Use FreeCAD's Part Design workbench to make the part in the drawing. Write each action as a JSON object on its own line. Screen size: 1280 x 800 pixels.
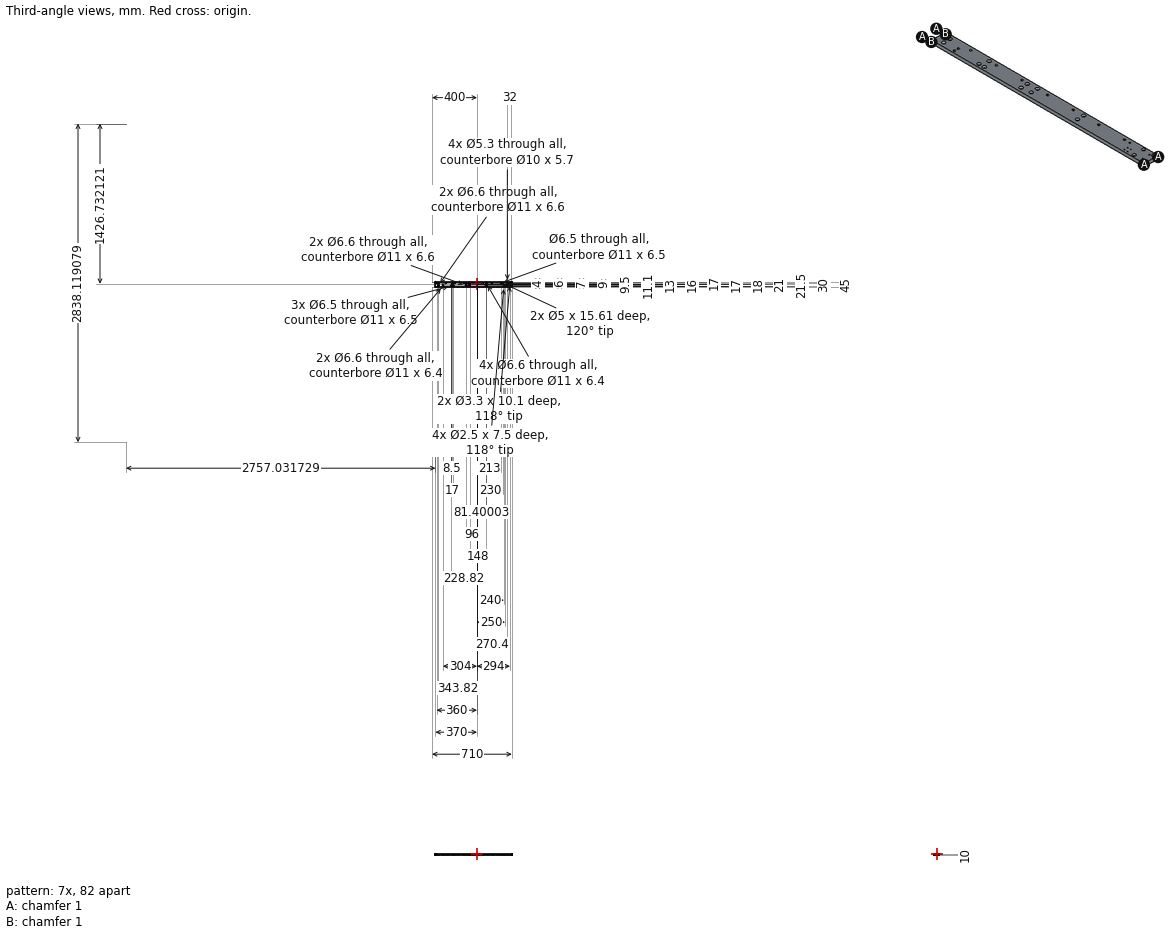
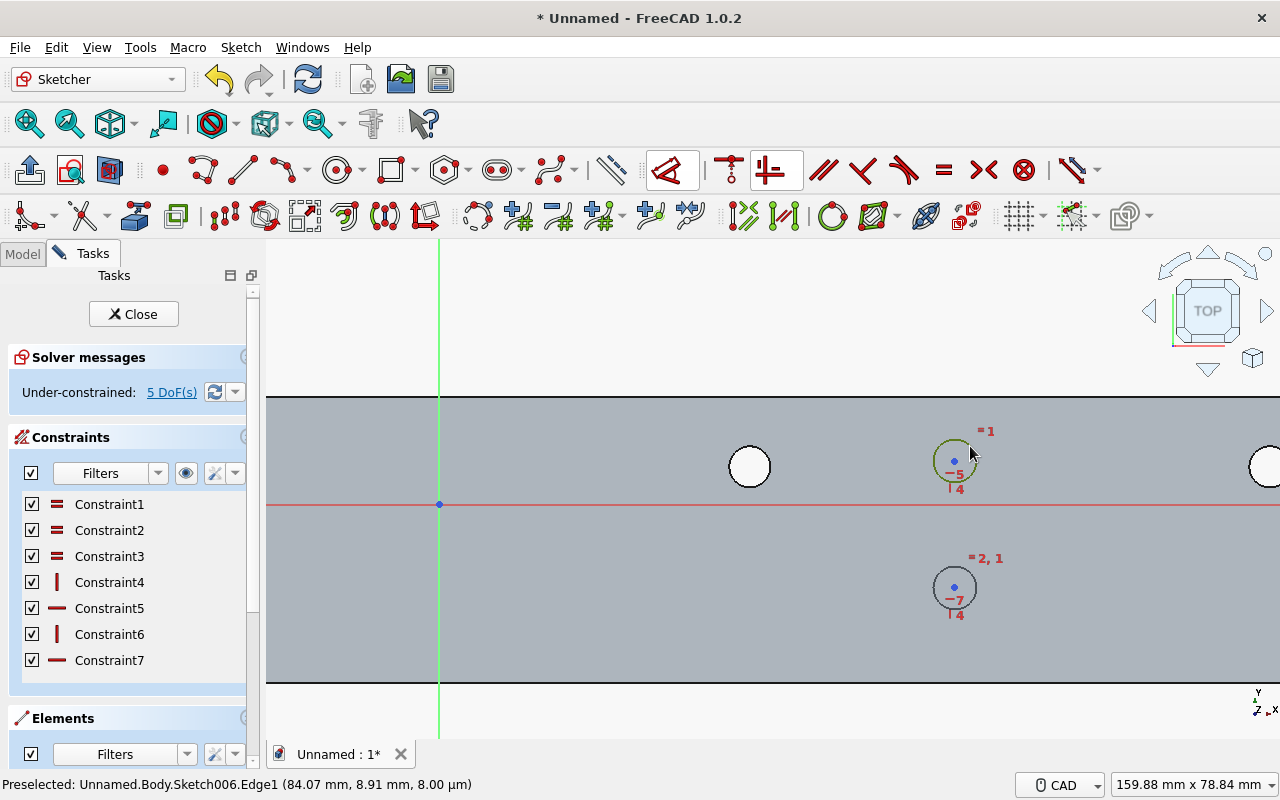
{"action": "left_click", "coordinate": [694, 170]}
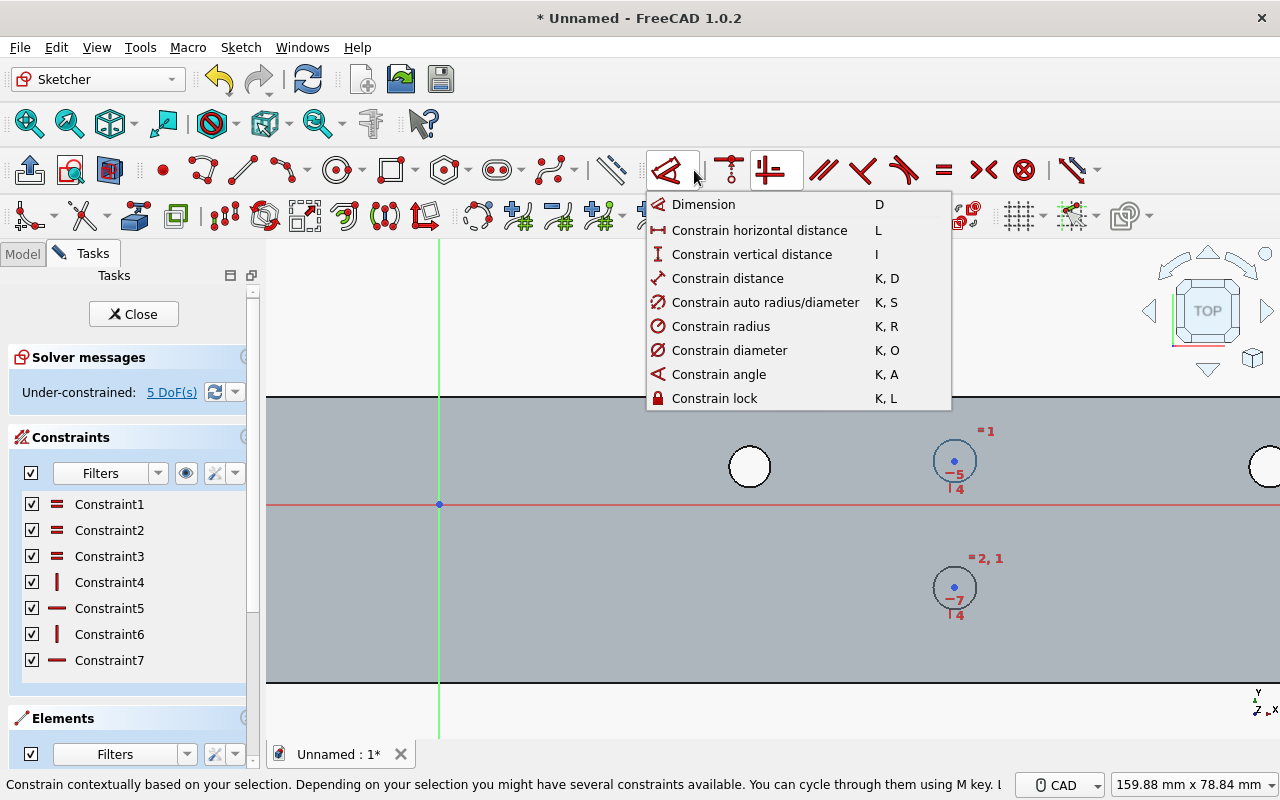
{"action": "left_click", "coordinate": [799, 350]}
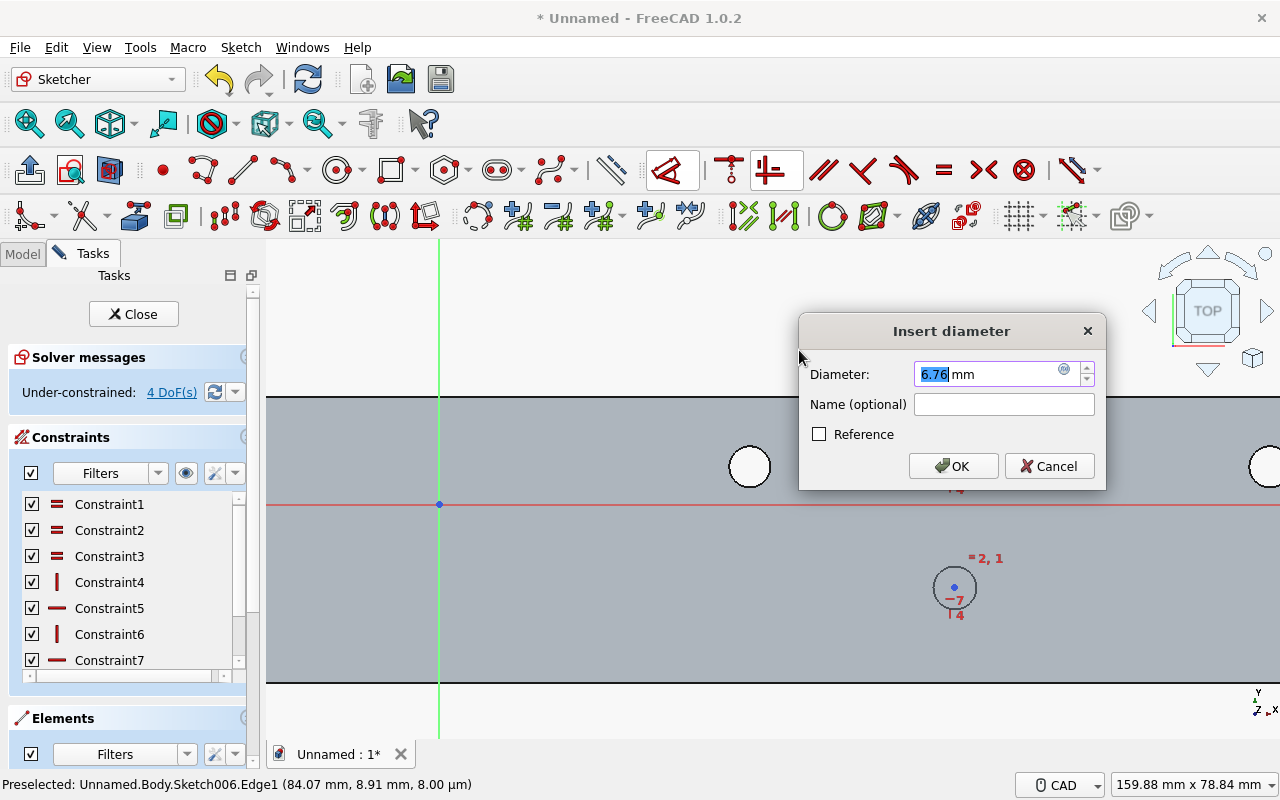
{"action": "type", "text": "6.6"}
{"action": "key", "text": "Return"}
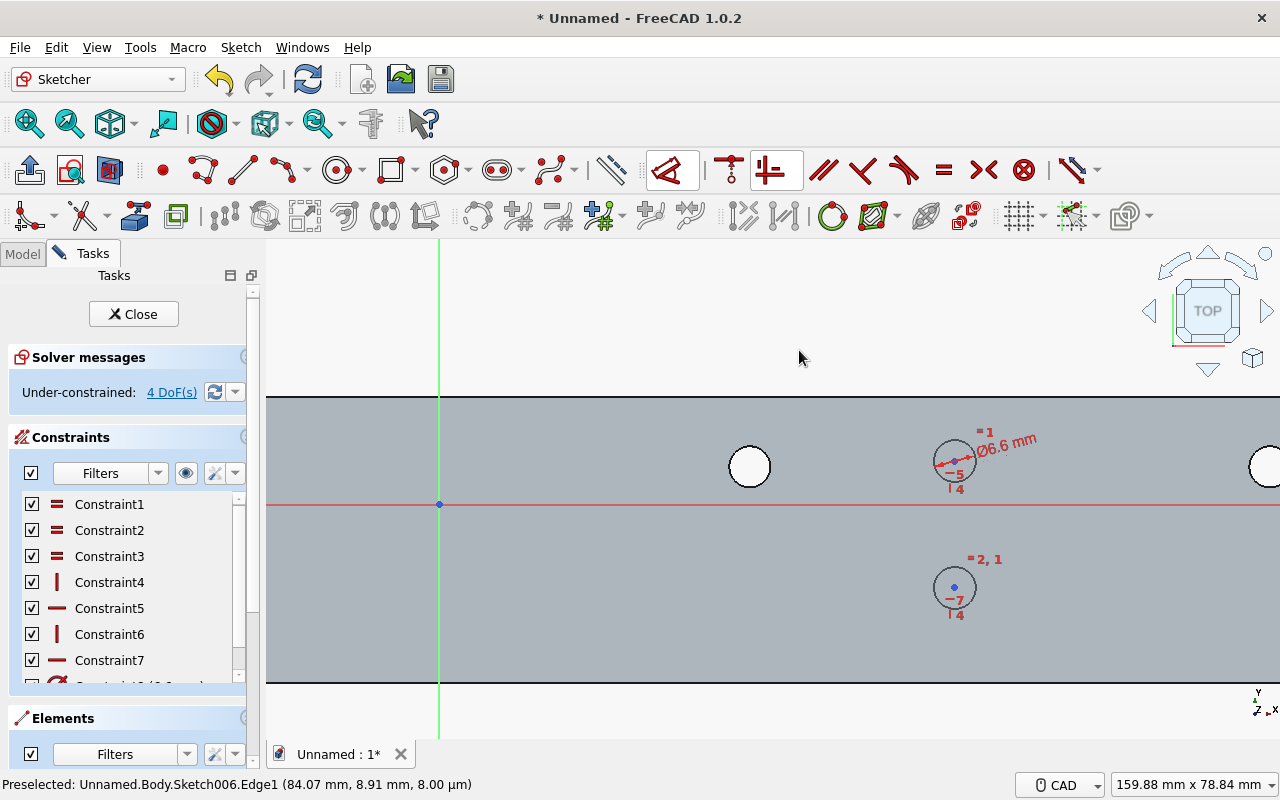
{"action": "left_click", "coordinate": [955, 461]}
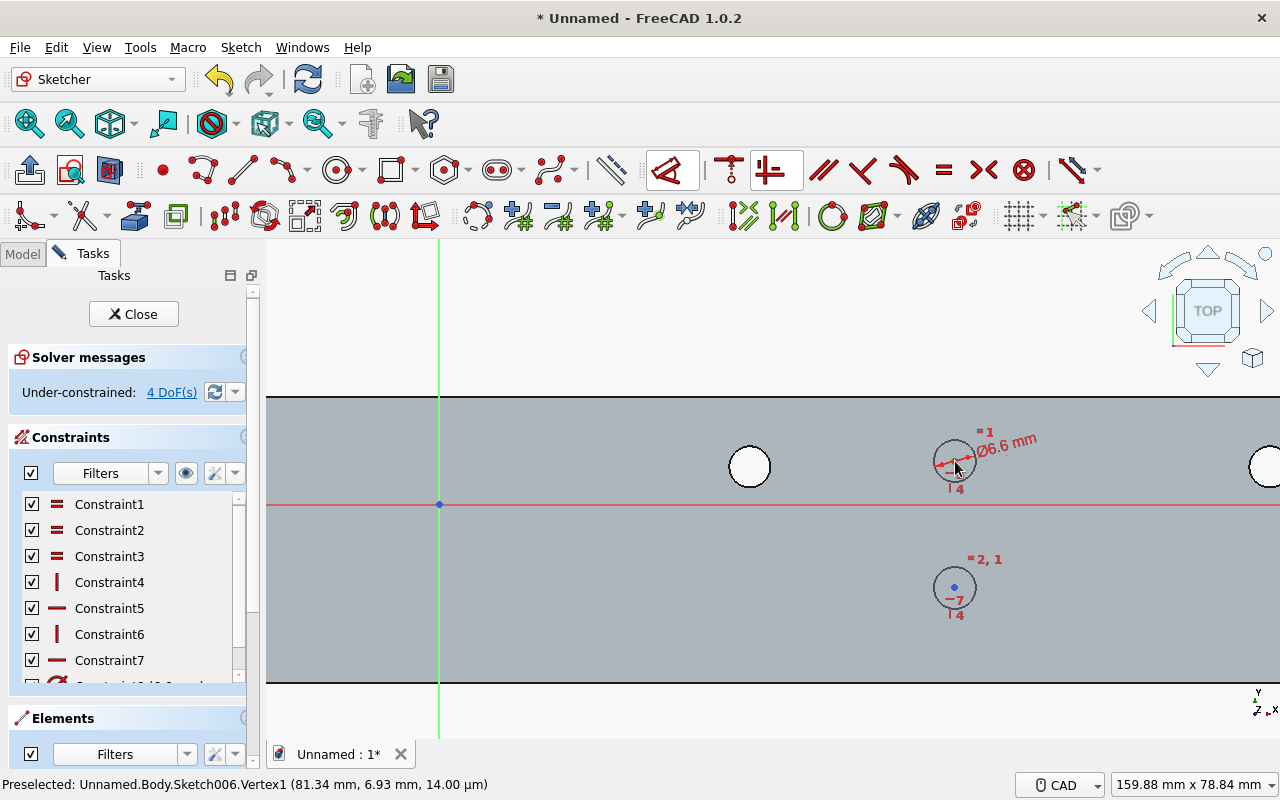
{"action": "key", "text": "i"}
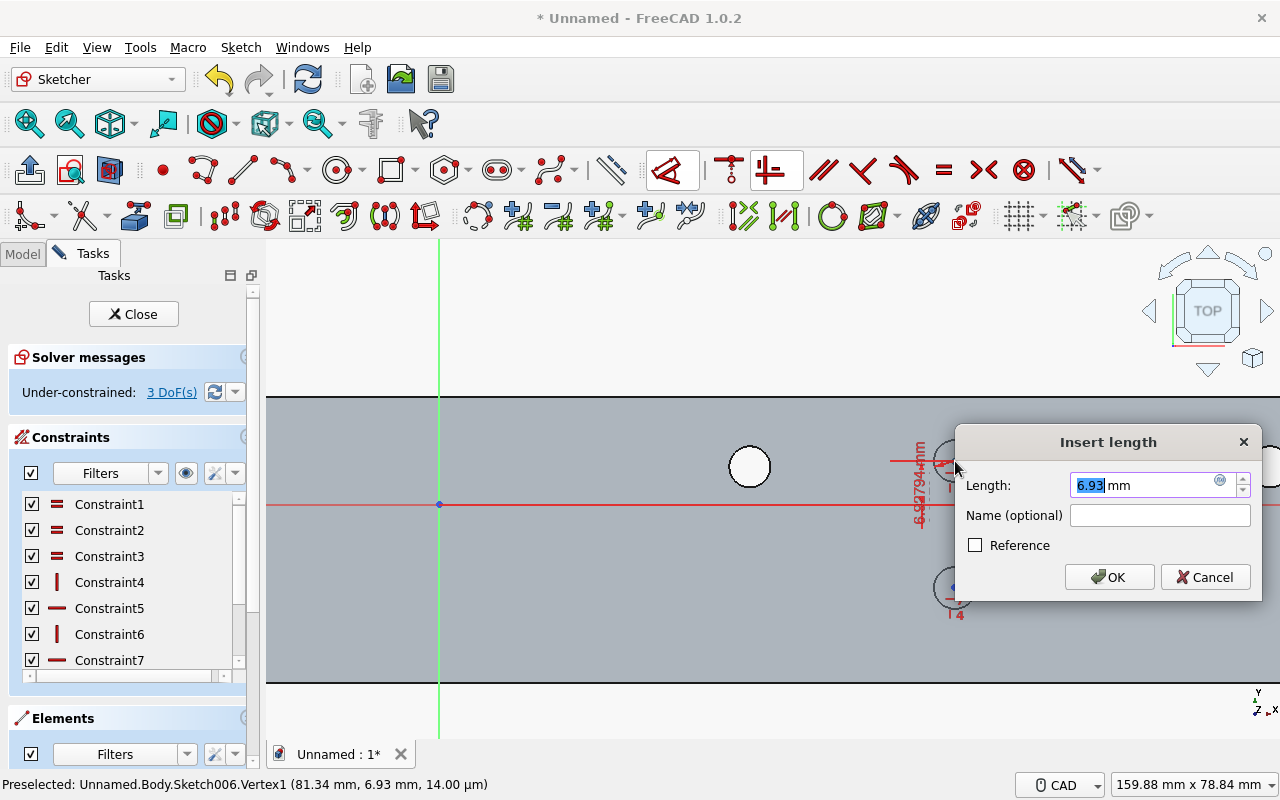
{"action": "type", "text": "7"}
{"action": "key", "text": "Return"}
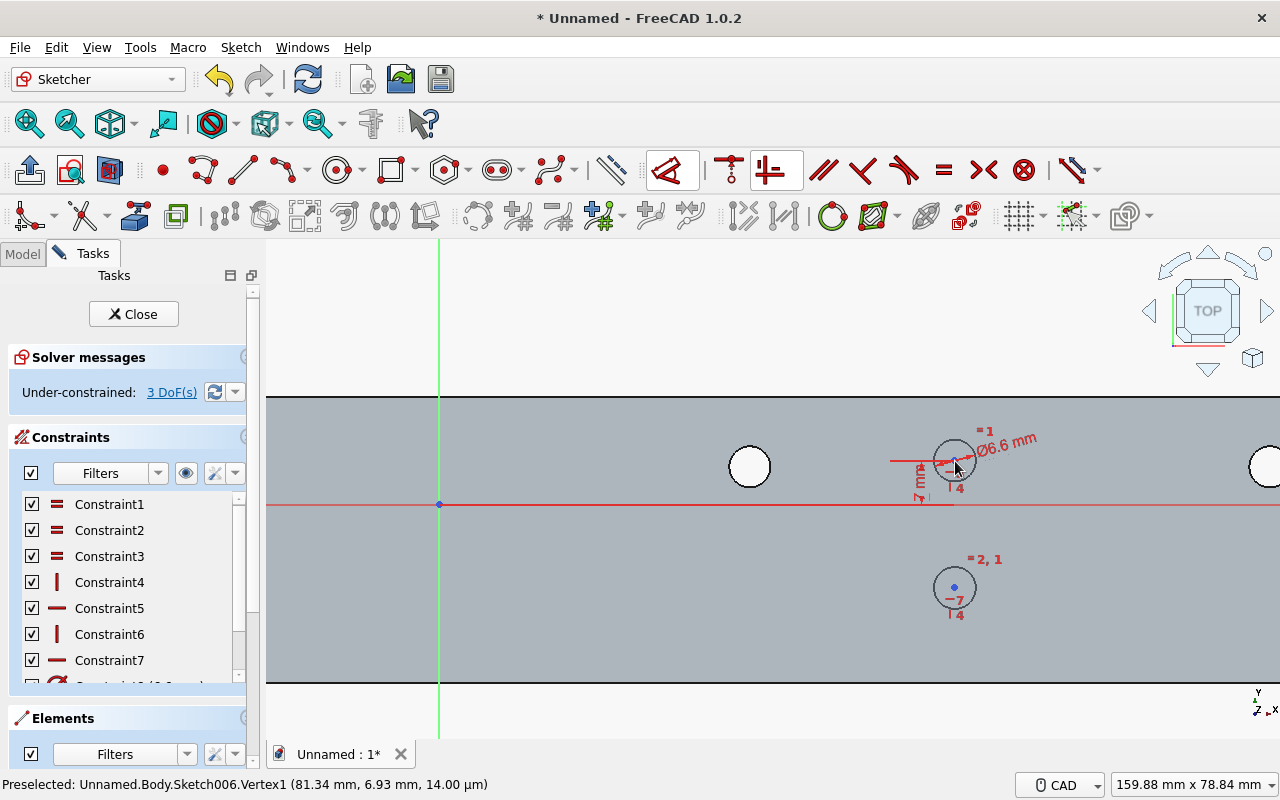
{"action": "left_click", "coordinate": [955, 588]}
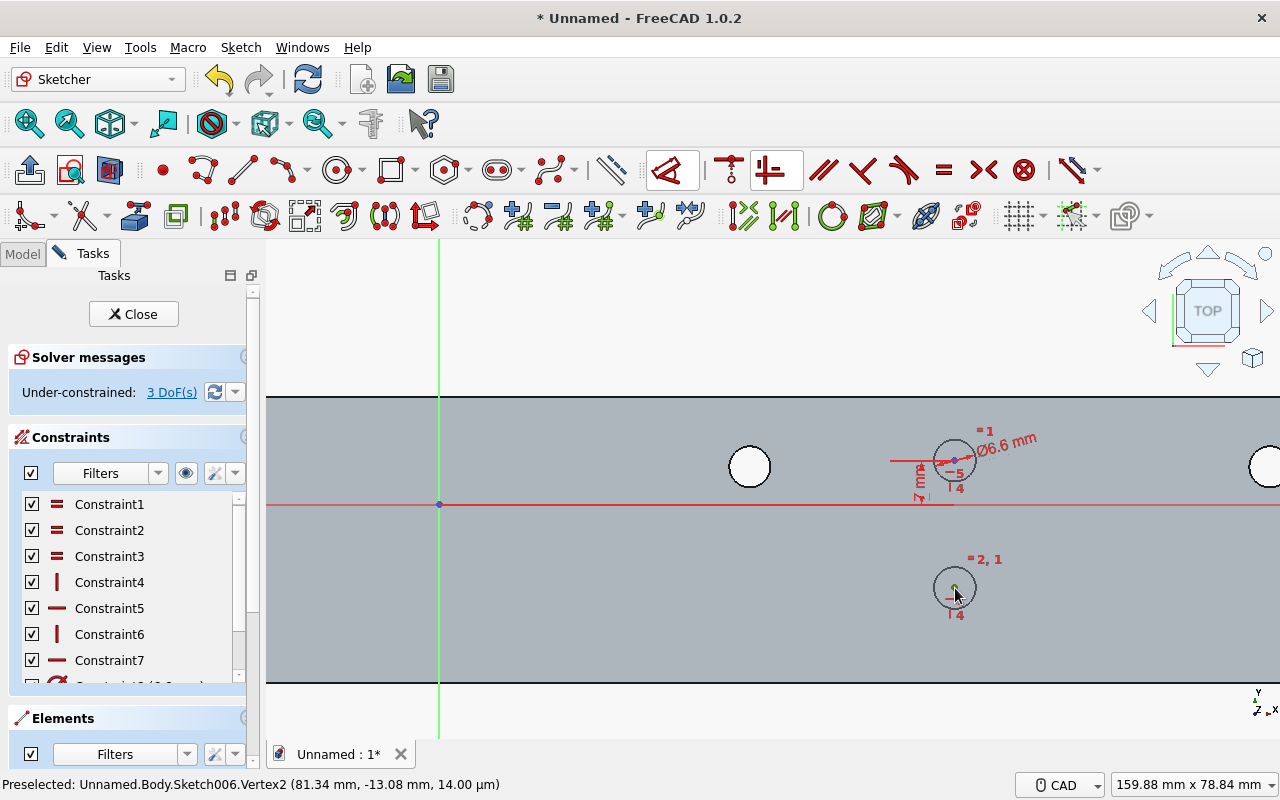
{"action": "left_click", "coordinate": [694, 170]}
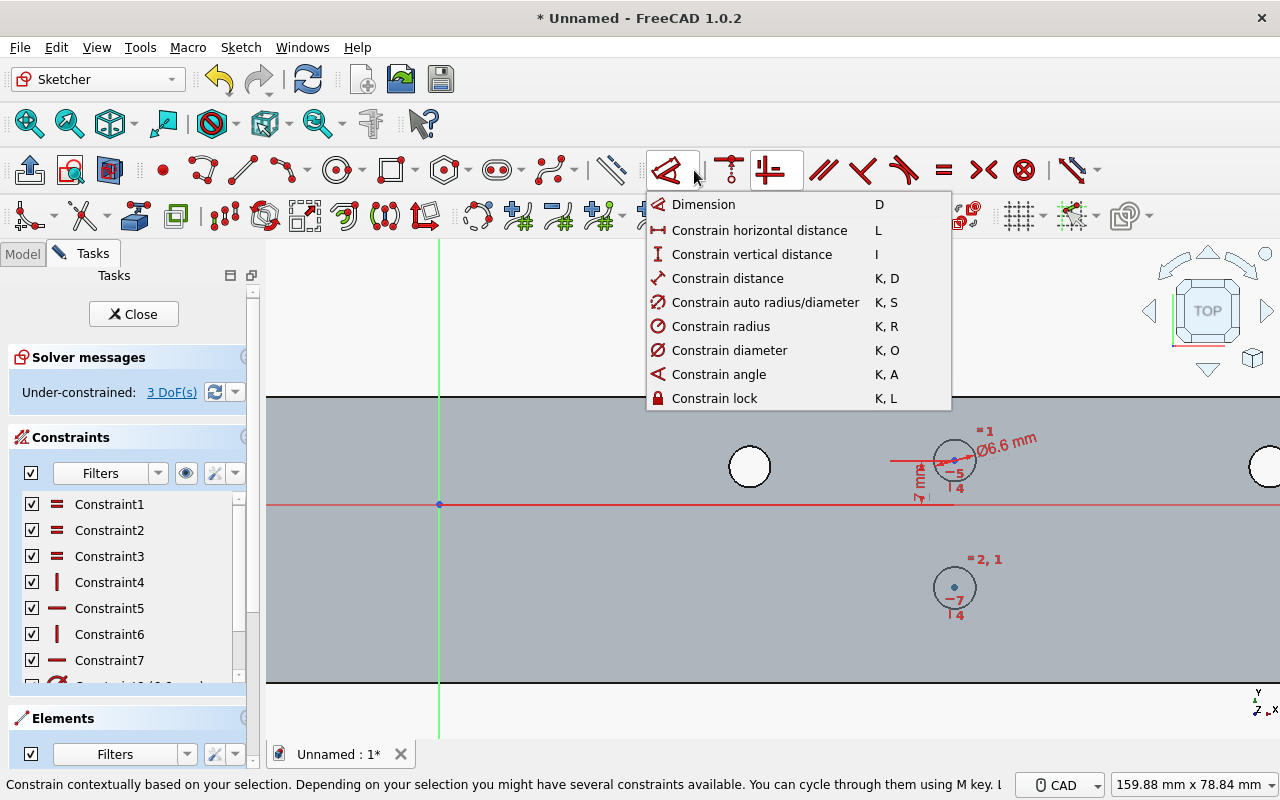
{"action": "left_click", "coordinate": [799, 254]}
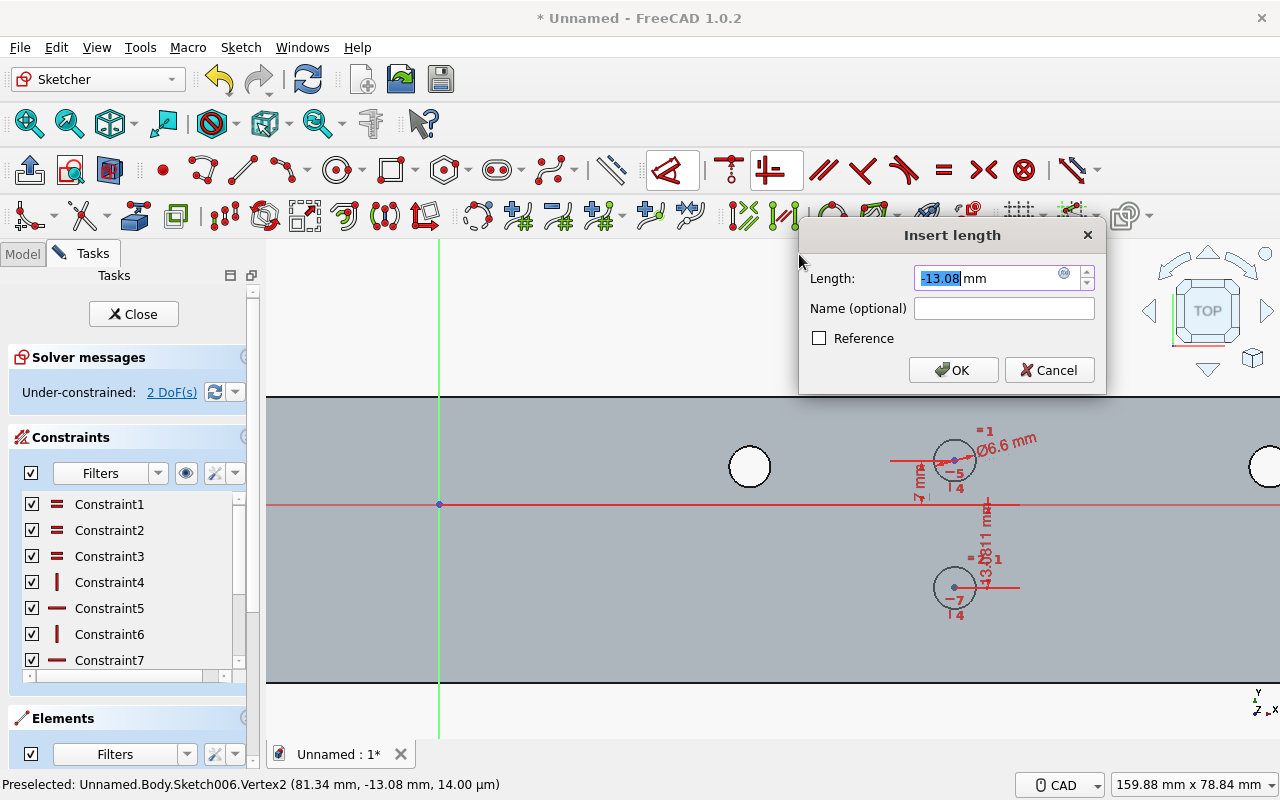
{"action": "type", "text": "-13"}
{"action": "key", "text": "Return"}